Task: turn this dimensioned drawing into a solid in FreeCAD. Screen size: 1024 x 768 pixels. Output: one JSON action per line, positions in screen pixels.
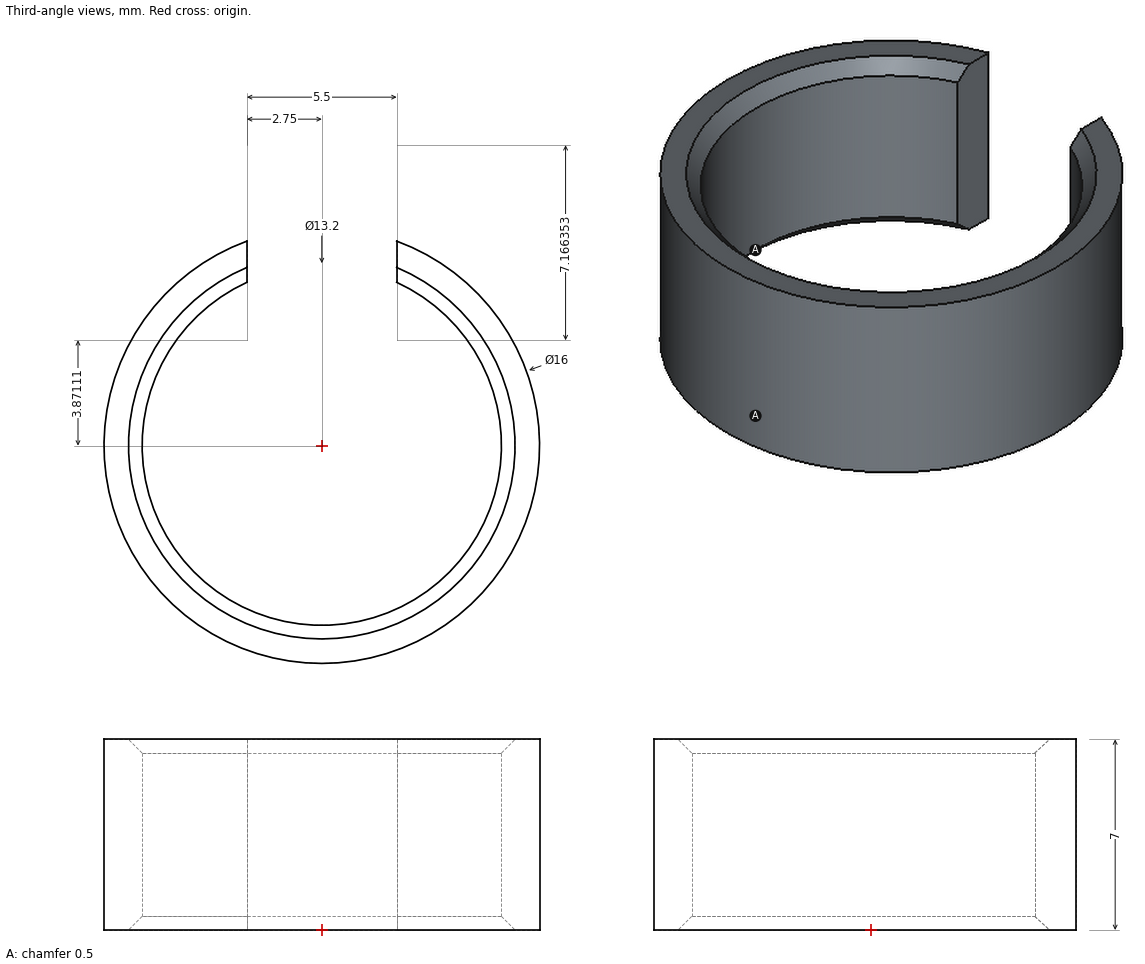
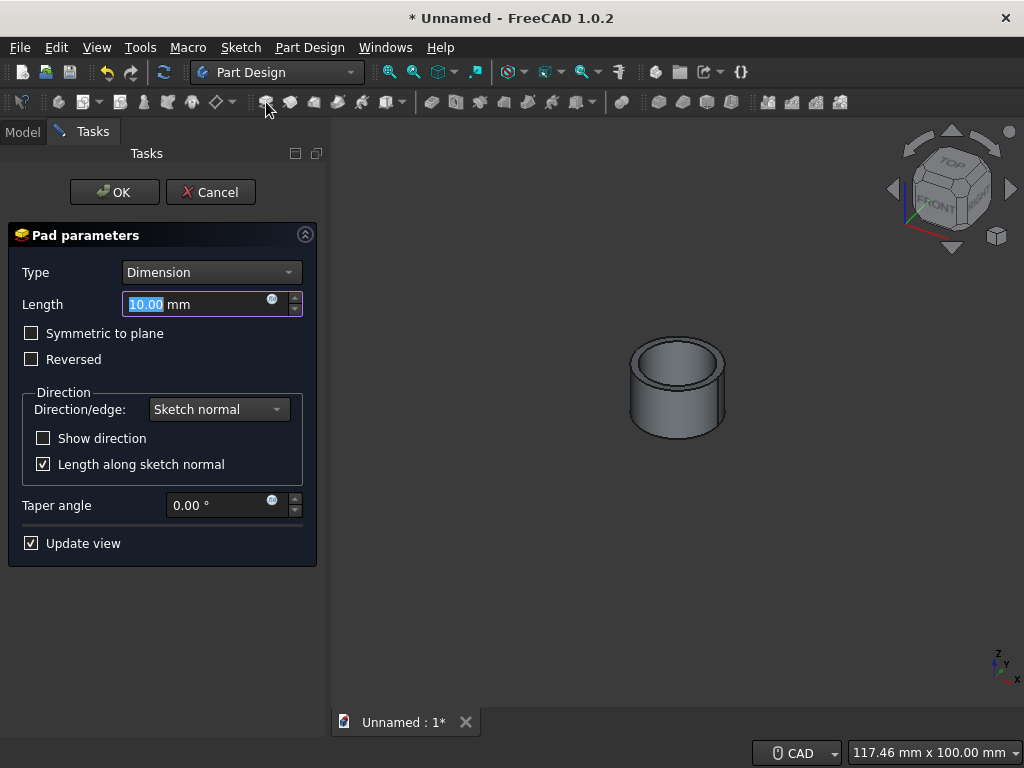
{"action": "type", "text": "7"}
{"action": "key", "text": "Tab"}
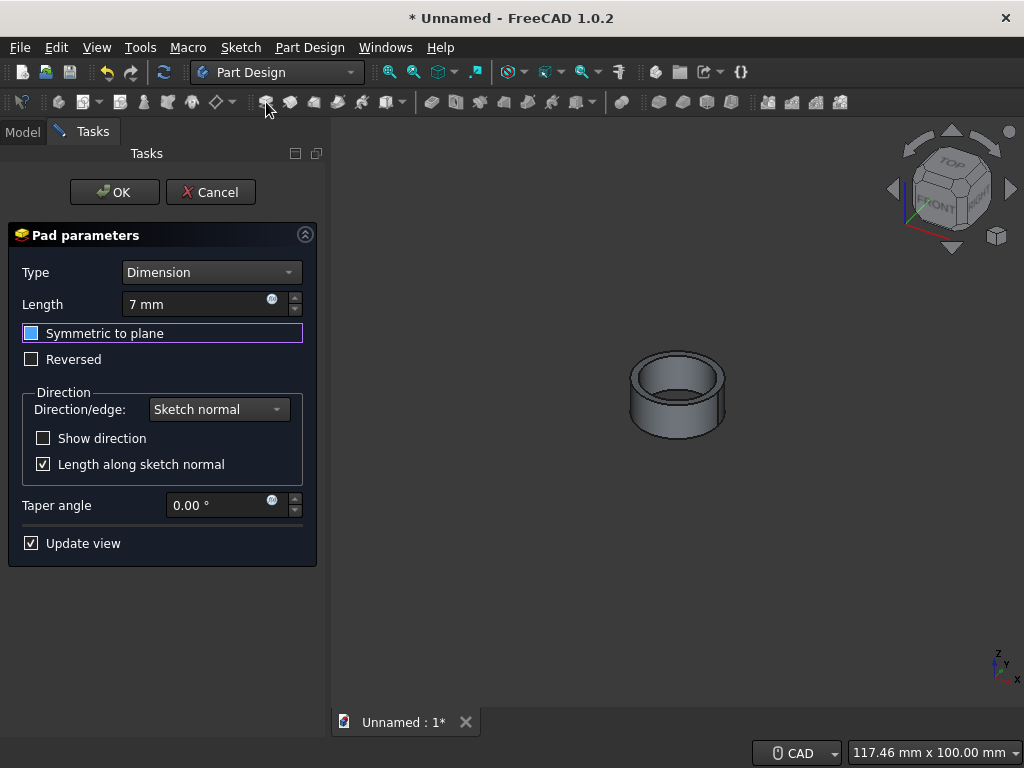
{"action": "left_click", "coordinate": [115, 192]}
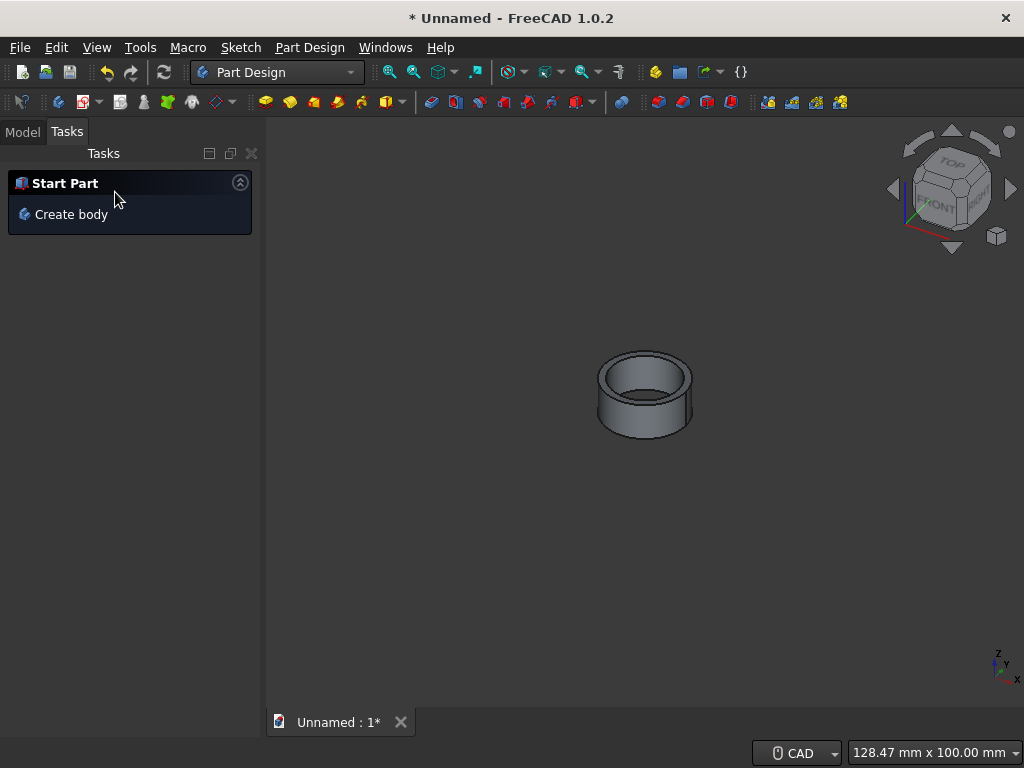
{"action": "left_click", "coordinate": [390, 72]}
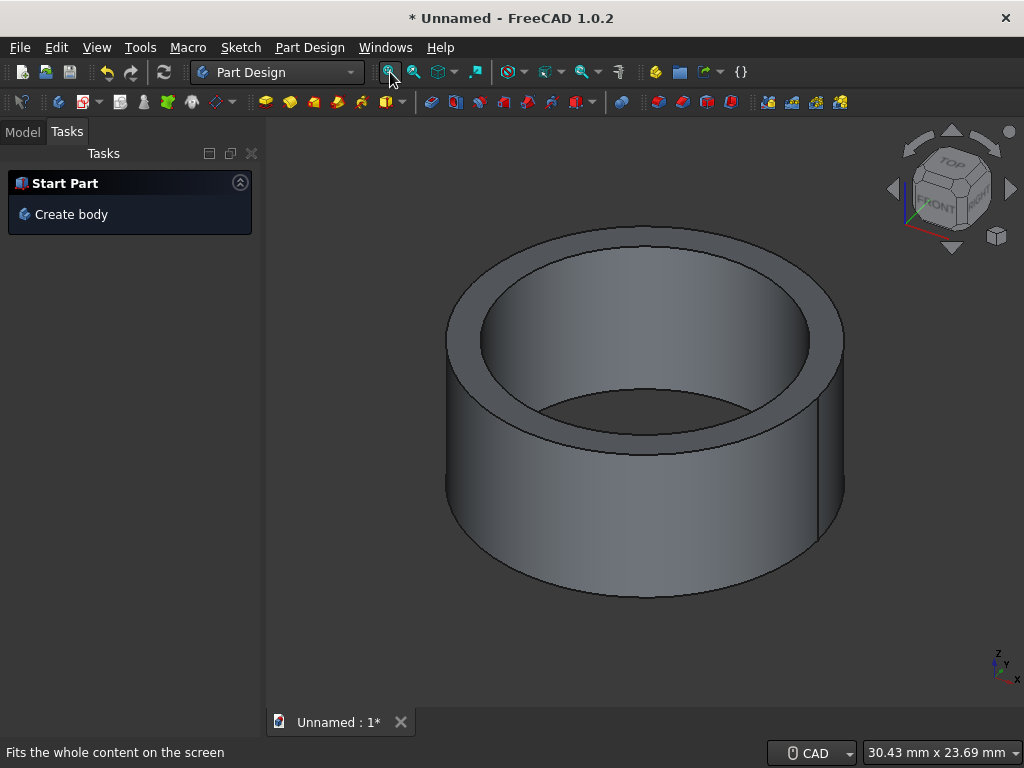
{"action": "left_click", "coordinate": [821, 360]}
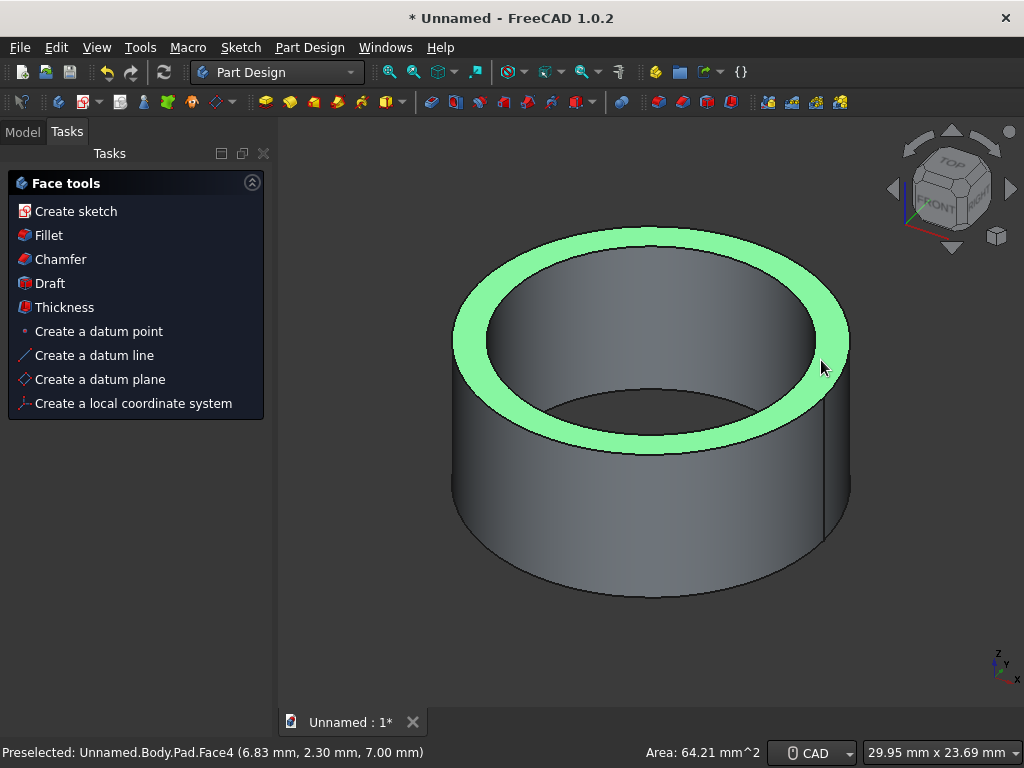
{"action": "left_click", "coordinate": [84, 102]}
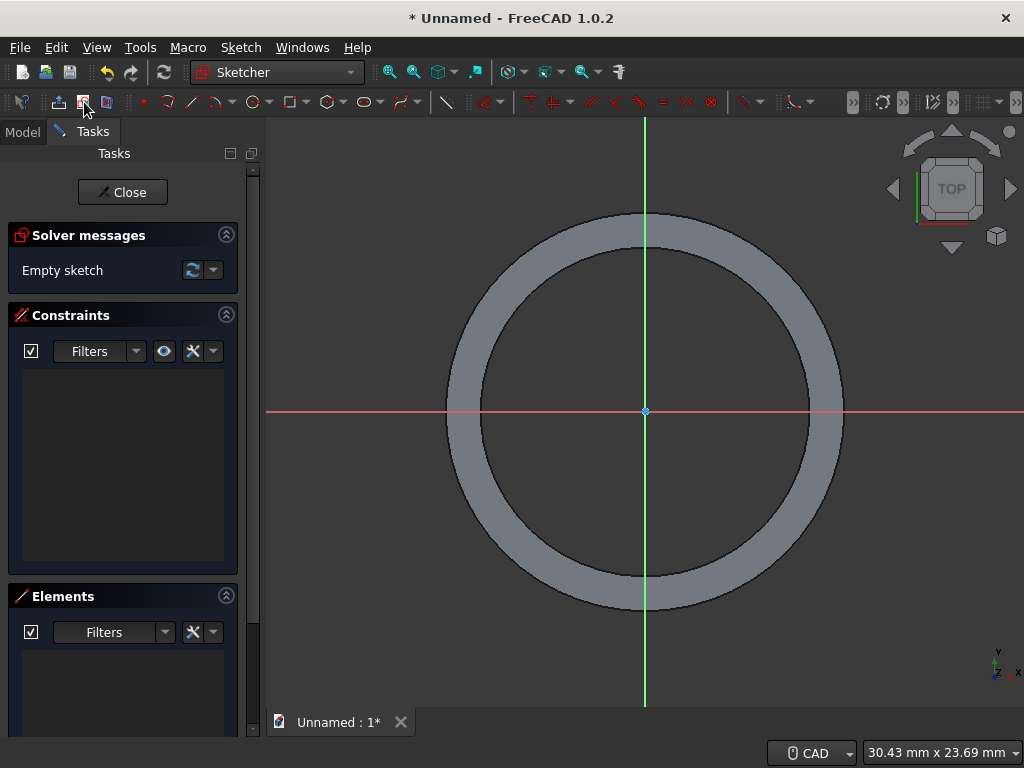
{"action": "scroll", "coordinate": [294, 679], "scroll_direction": "down", "scroll_amount": 1}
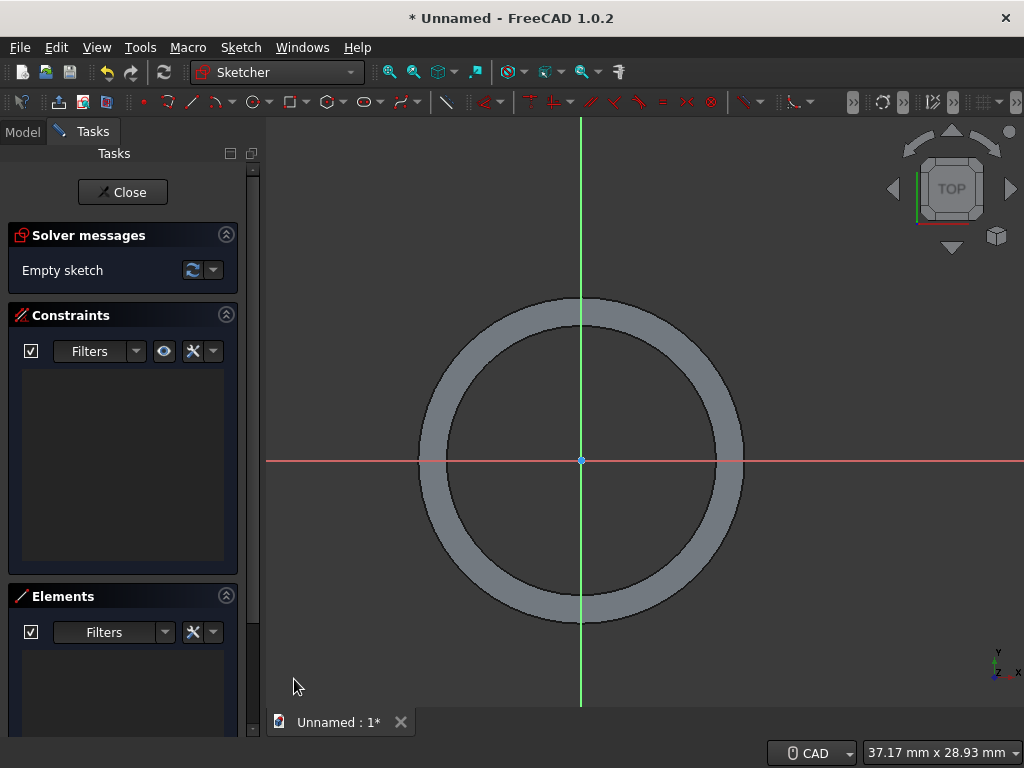
{"action": "scroll", "coordinate": [587, 270], "scroll_direction": "up", "scroll_amount": 3}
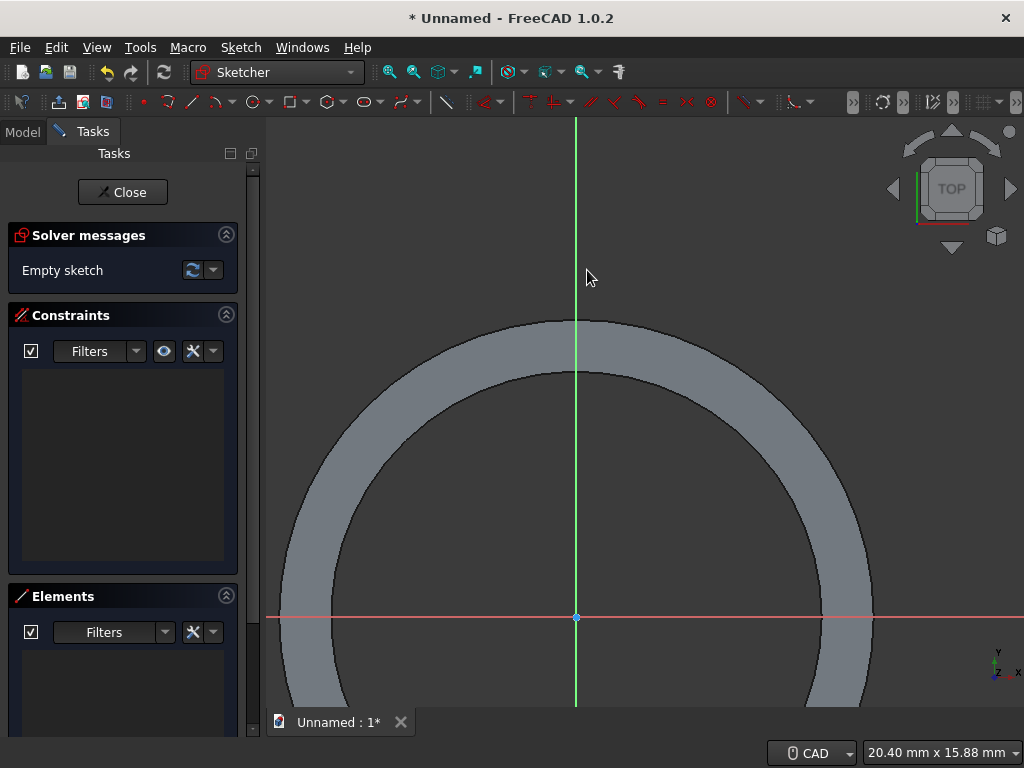
{"action": "left_click", "coordinate": [290, 102]}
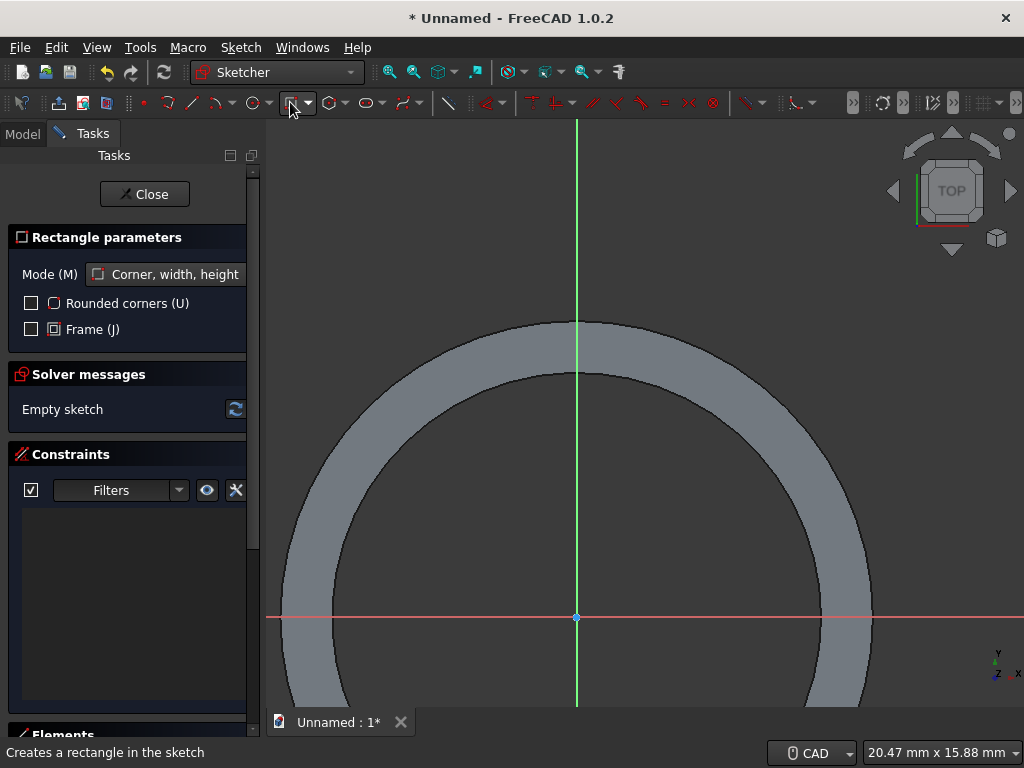
{"action": "left_click", "coordinate": [475, 209]}
{"action": "mouse_move", "coordinate": [678, 474]}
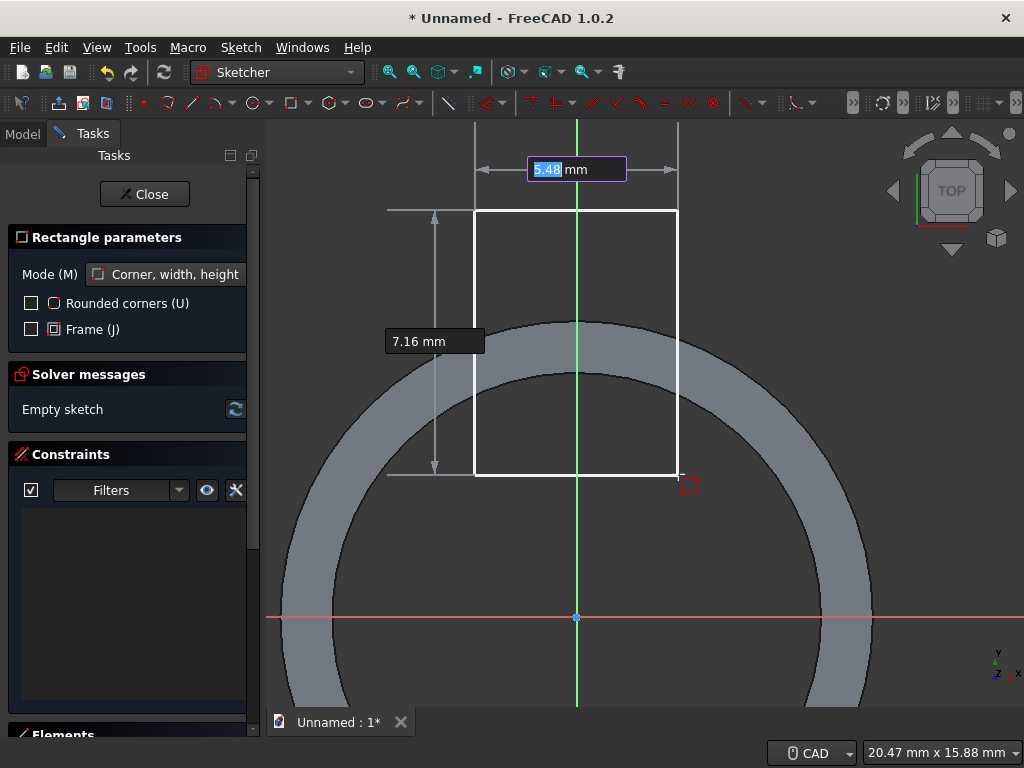
{"action": "type", "text": "5.5"}
{"action": "key", "text": "Tab"}
{"action": "type", "text": "7.166353"}
{"action": "key", "text": "Return"}
{"action": "key", "text": "Escape"}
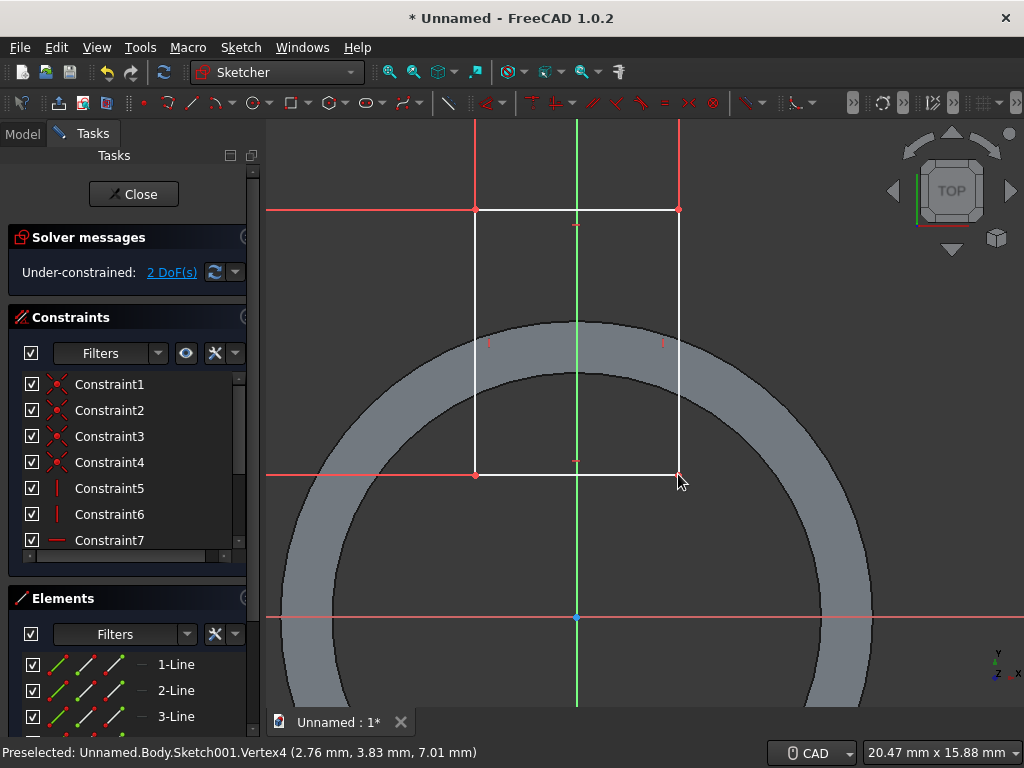
{"action": "left_click", "coordinate": [475, 210]}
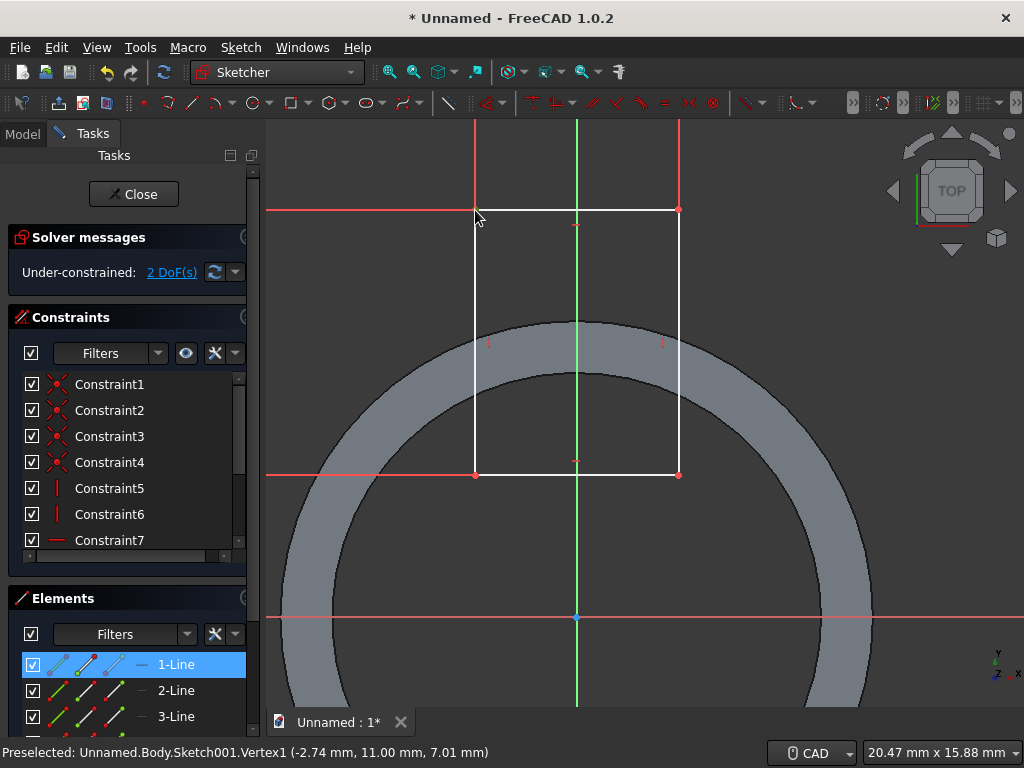
{"action": "key", "text": "l"}